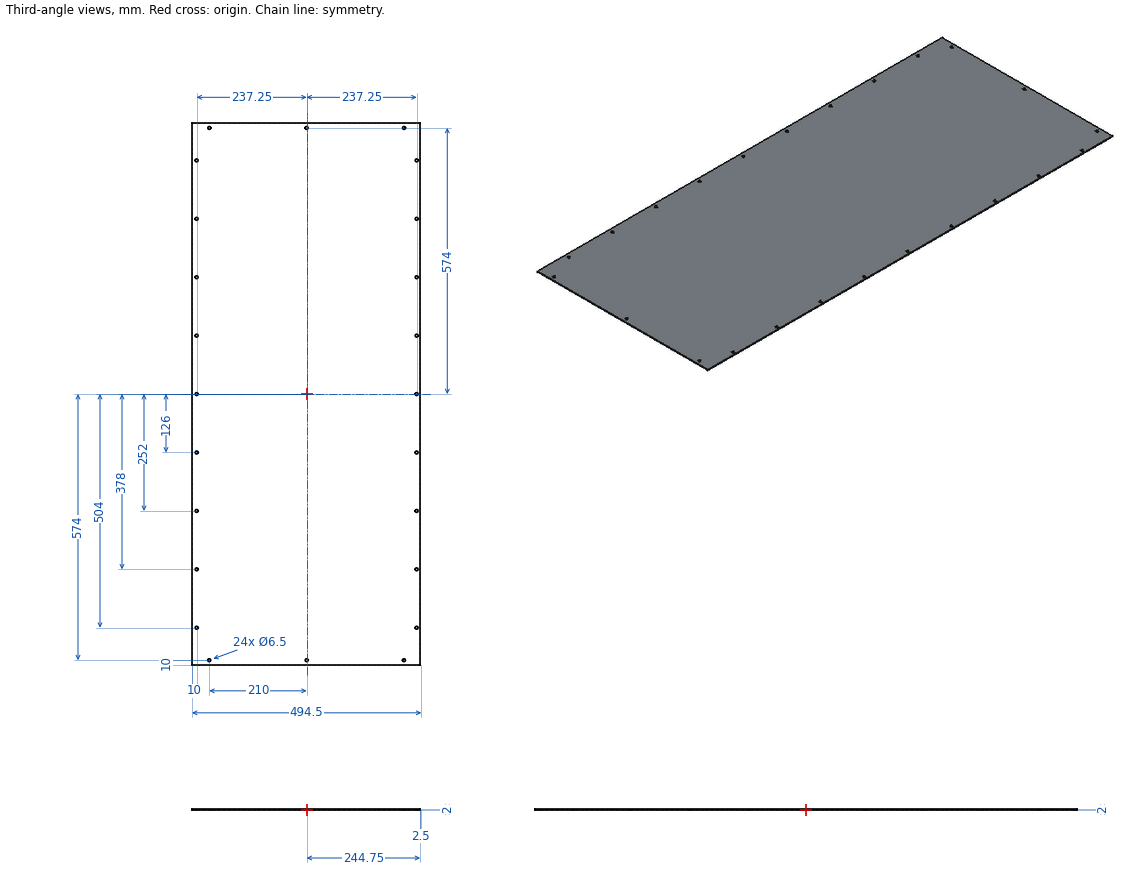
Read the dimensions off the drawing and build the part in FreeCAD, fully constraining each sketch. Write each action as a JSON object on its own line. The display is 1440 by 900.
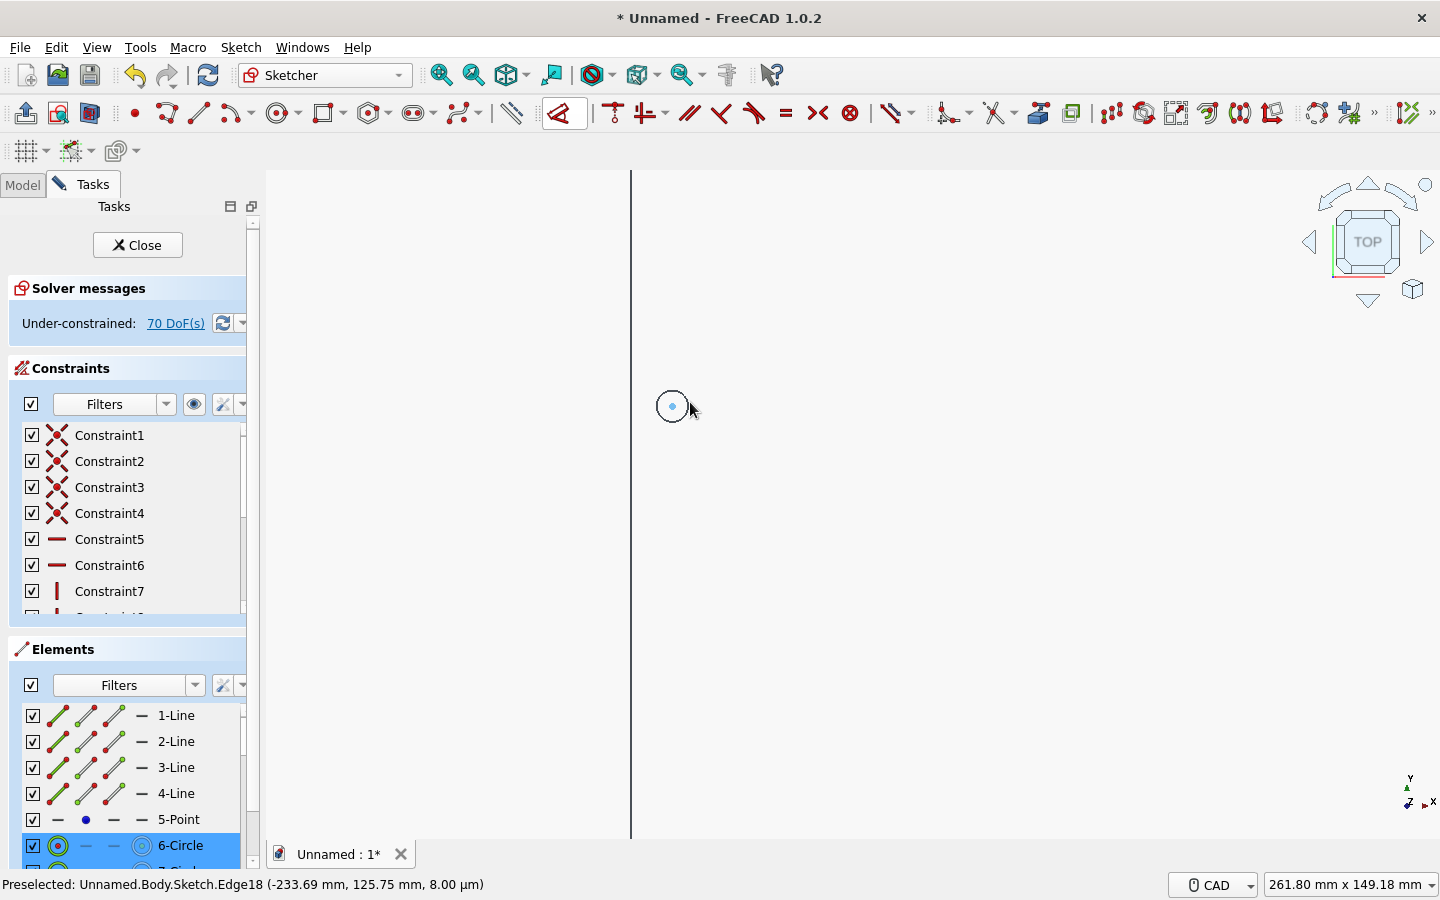
{"action": "left_click", "coordinate": [683, 395]}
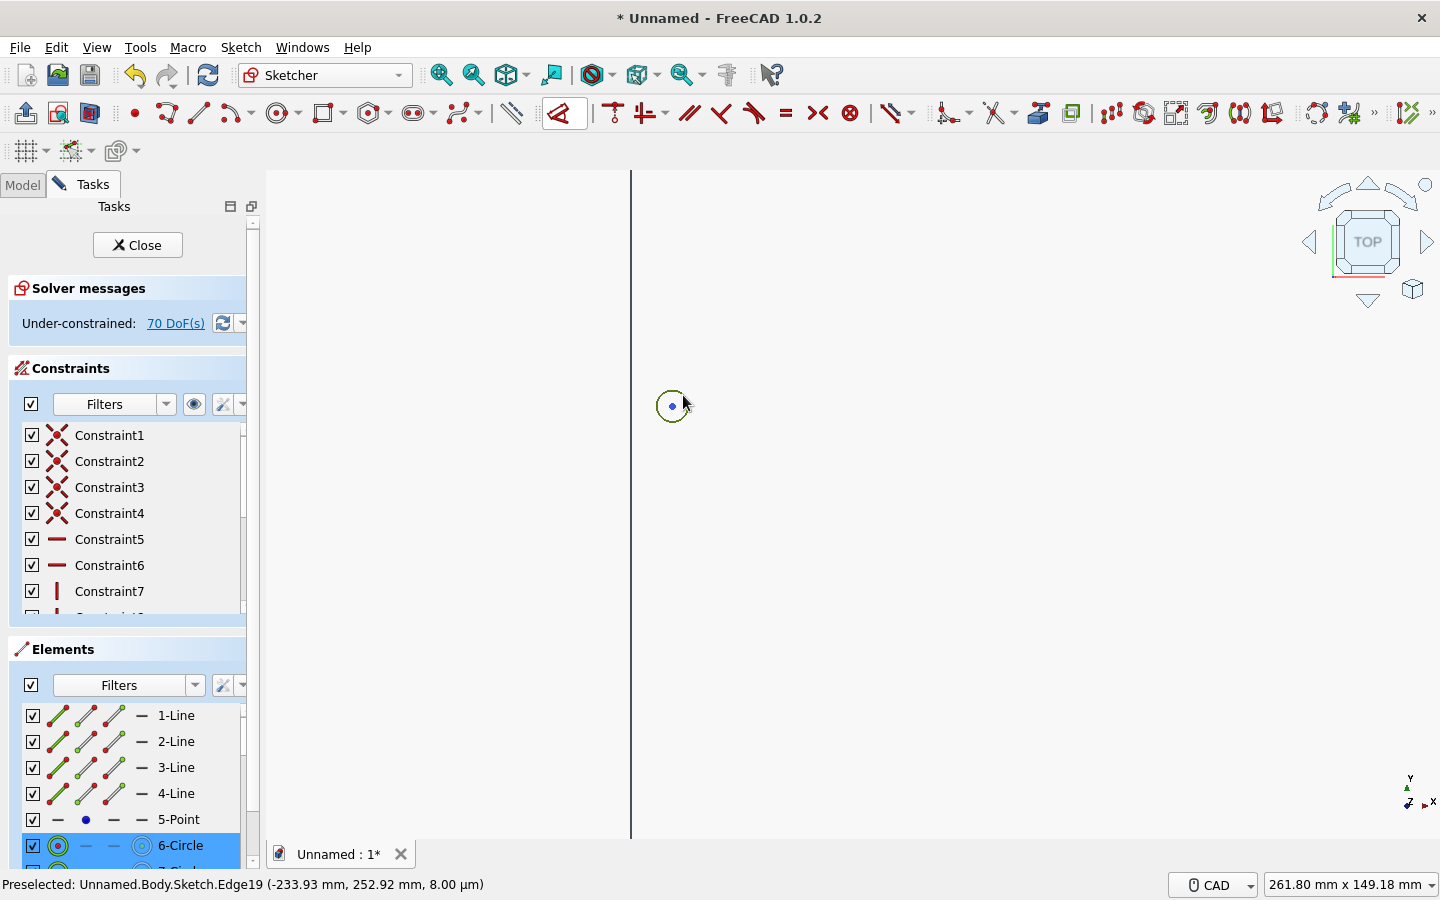
{"action": "scroll", "coordinate": [690, 402], "scroll_direction": "down", "scroll_amount": 12}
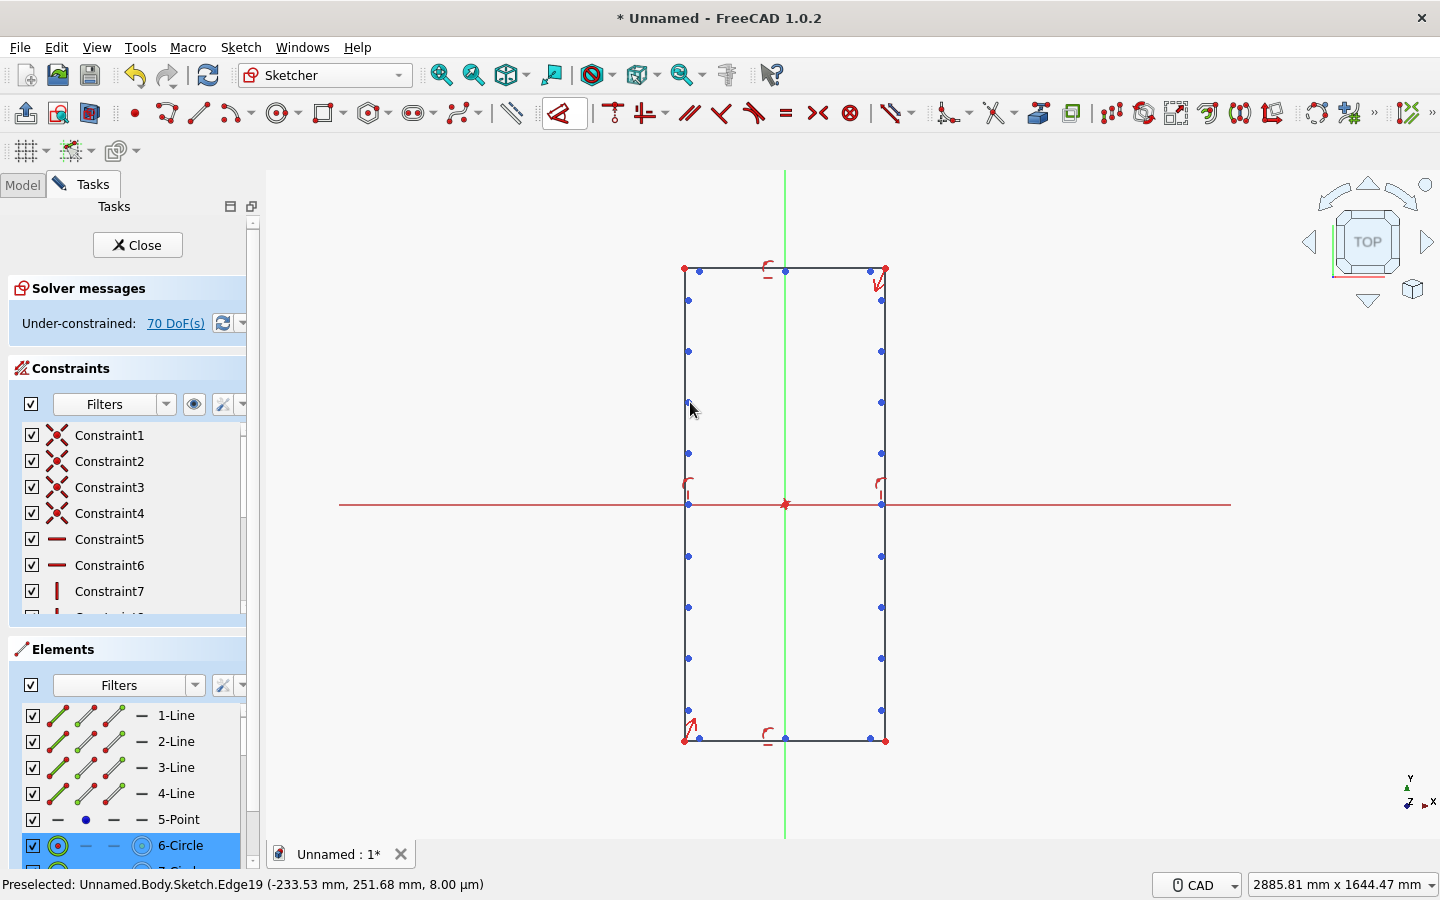
{"action": "scroll", "coordinate": [690, 350], "scroll_direction": "up", "scroll_amount": 11}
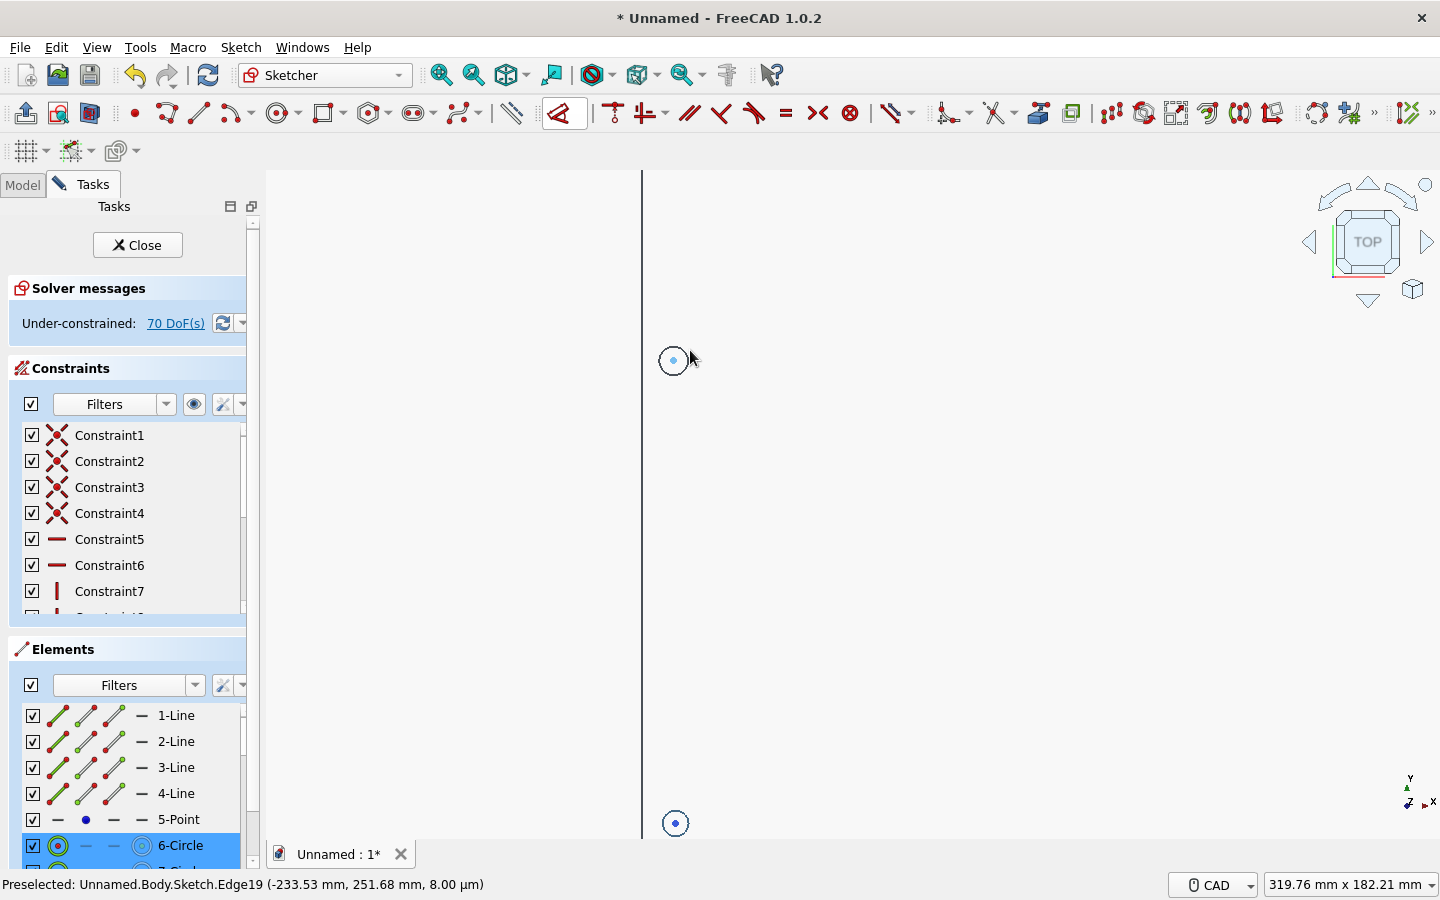
{"action": "left_click", "coordinate": [684, 351]}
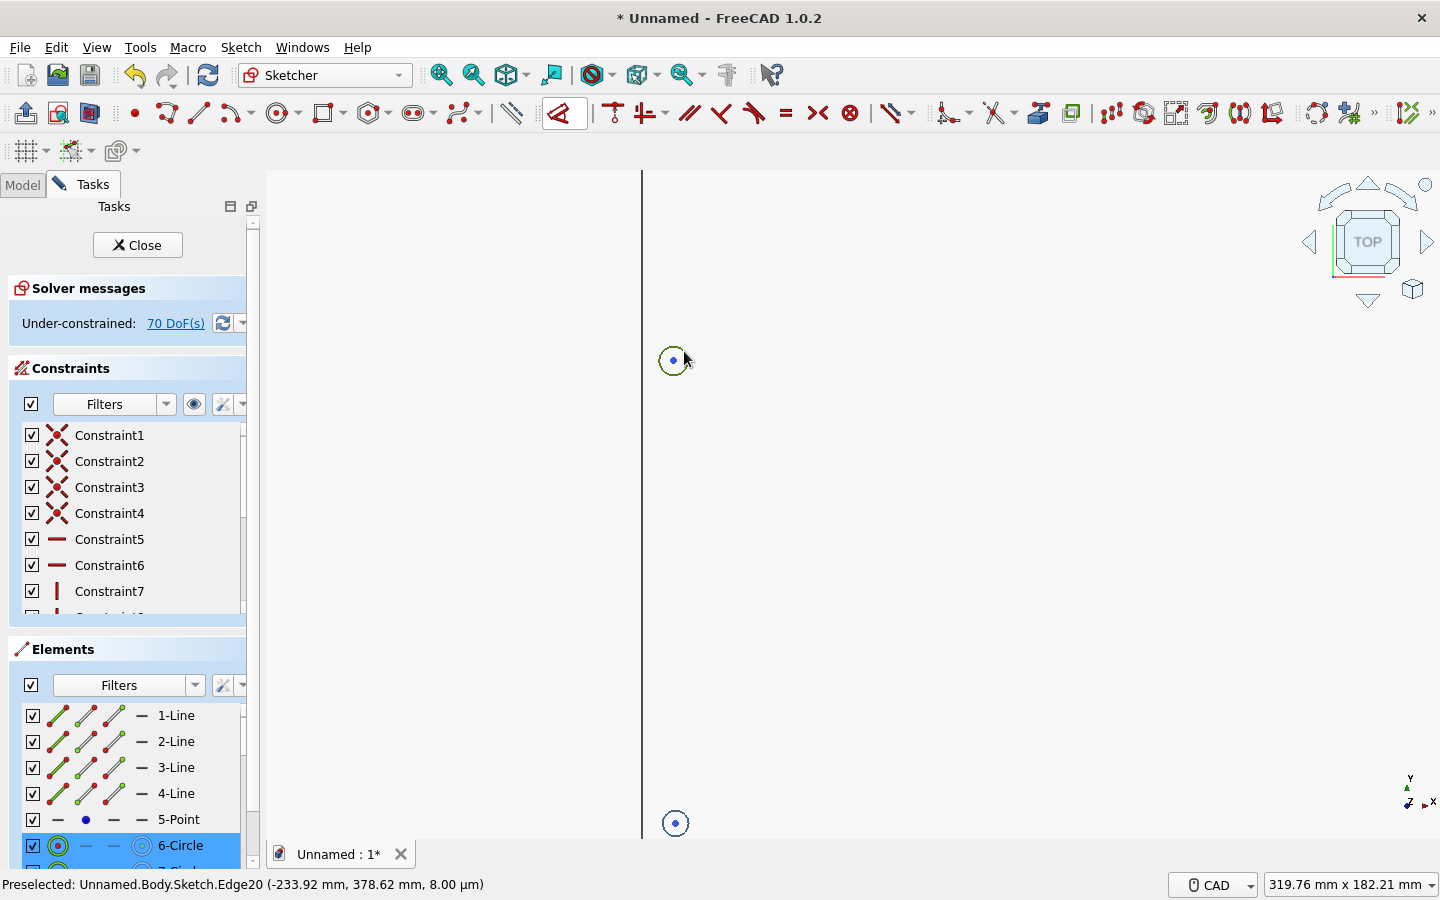
{"action": "scroll", "coordinate": [690, 350], "scroll_direction": "down", "scroll_amount": 11}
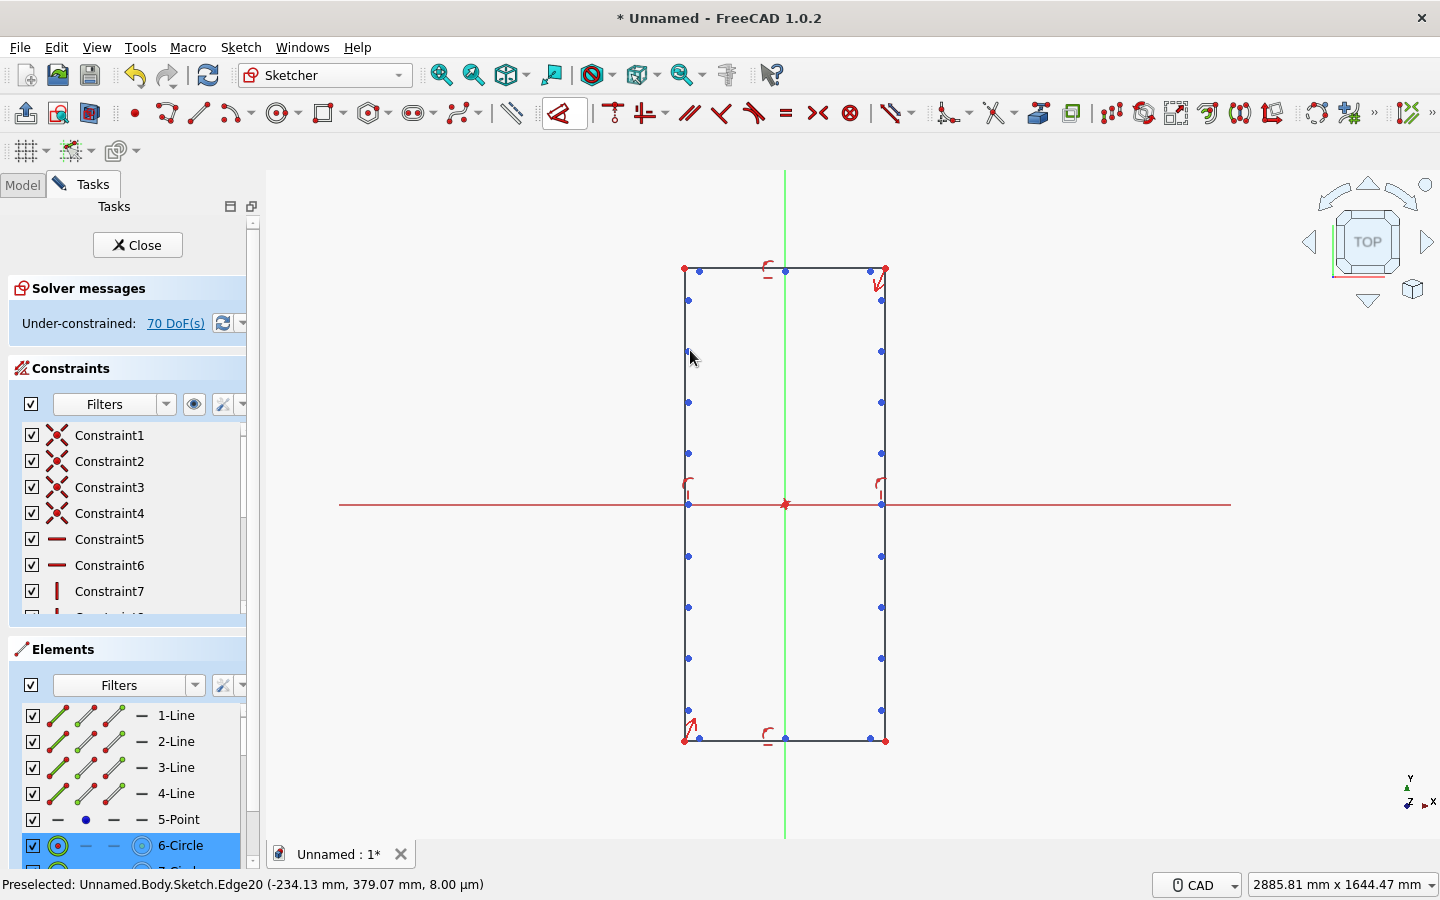
{"action": "scroll", "coordinate": [690, 299], "scroll_direction": "up", "scroll_amount": 12}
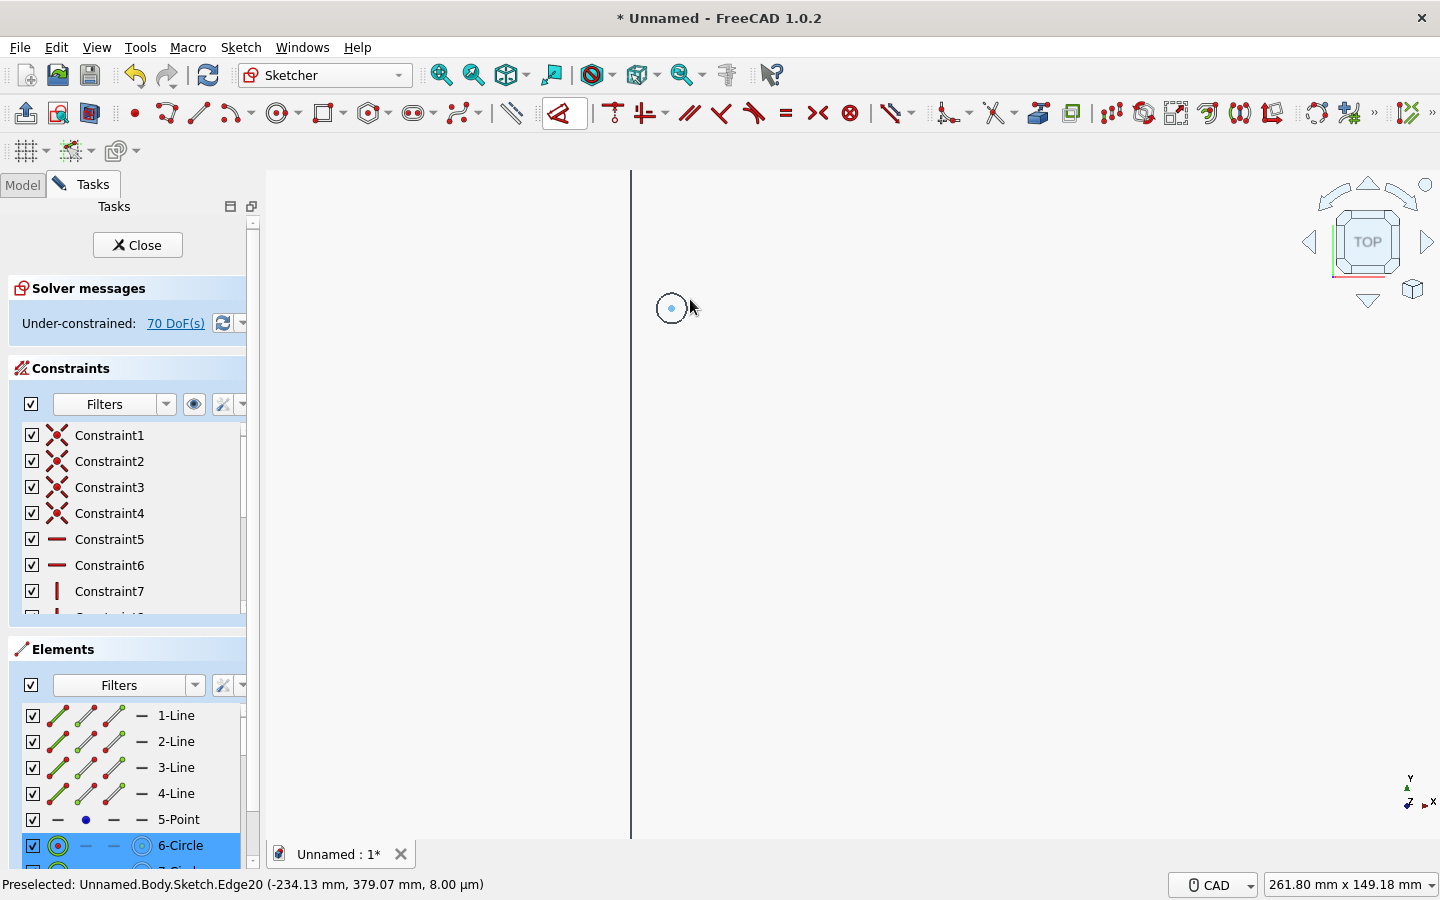
{"action": "left_click", "coordinate": [682, 298]}